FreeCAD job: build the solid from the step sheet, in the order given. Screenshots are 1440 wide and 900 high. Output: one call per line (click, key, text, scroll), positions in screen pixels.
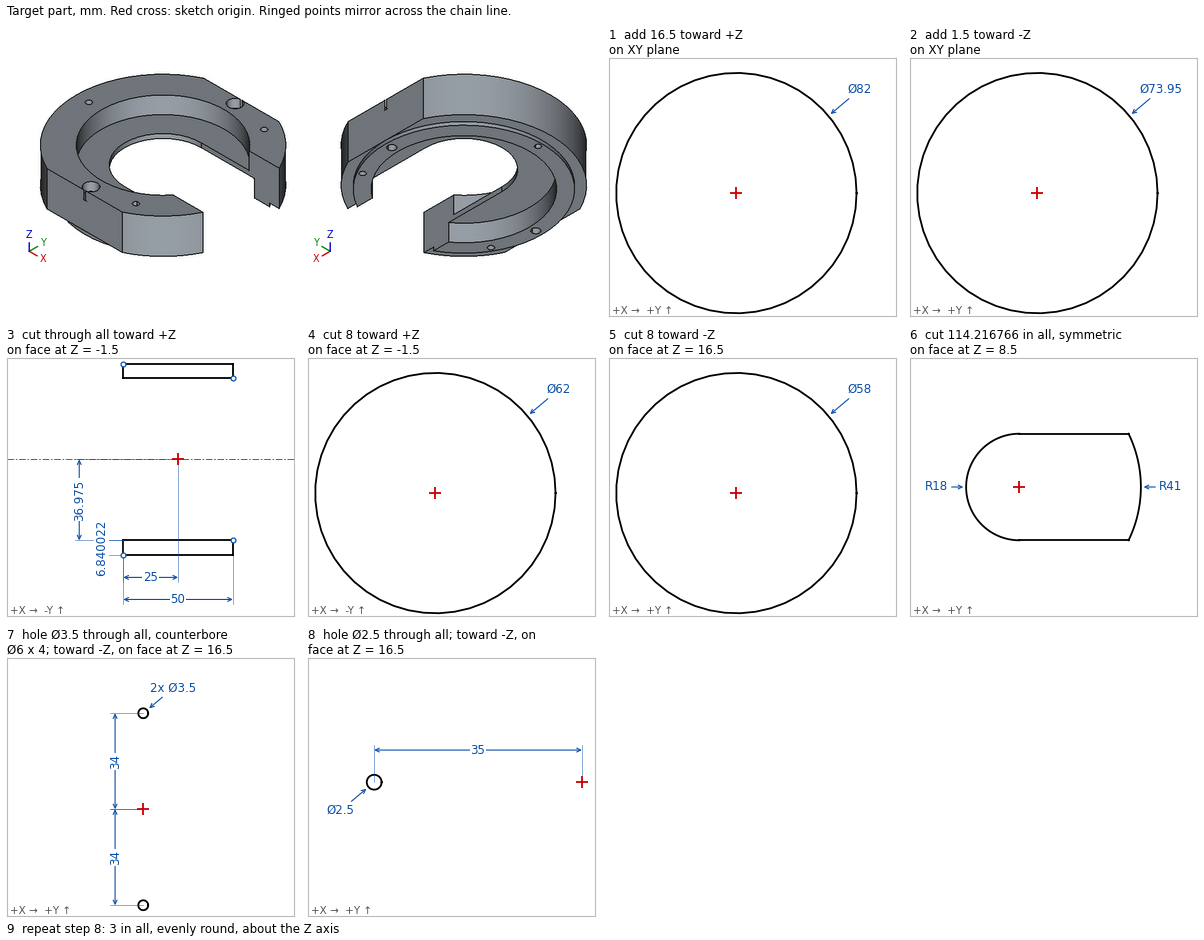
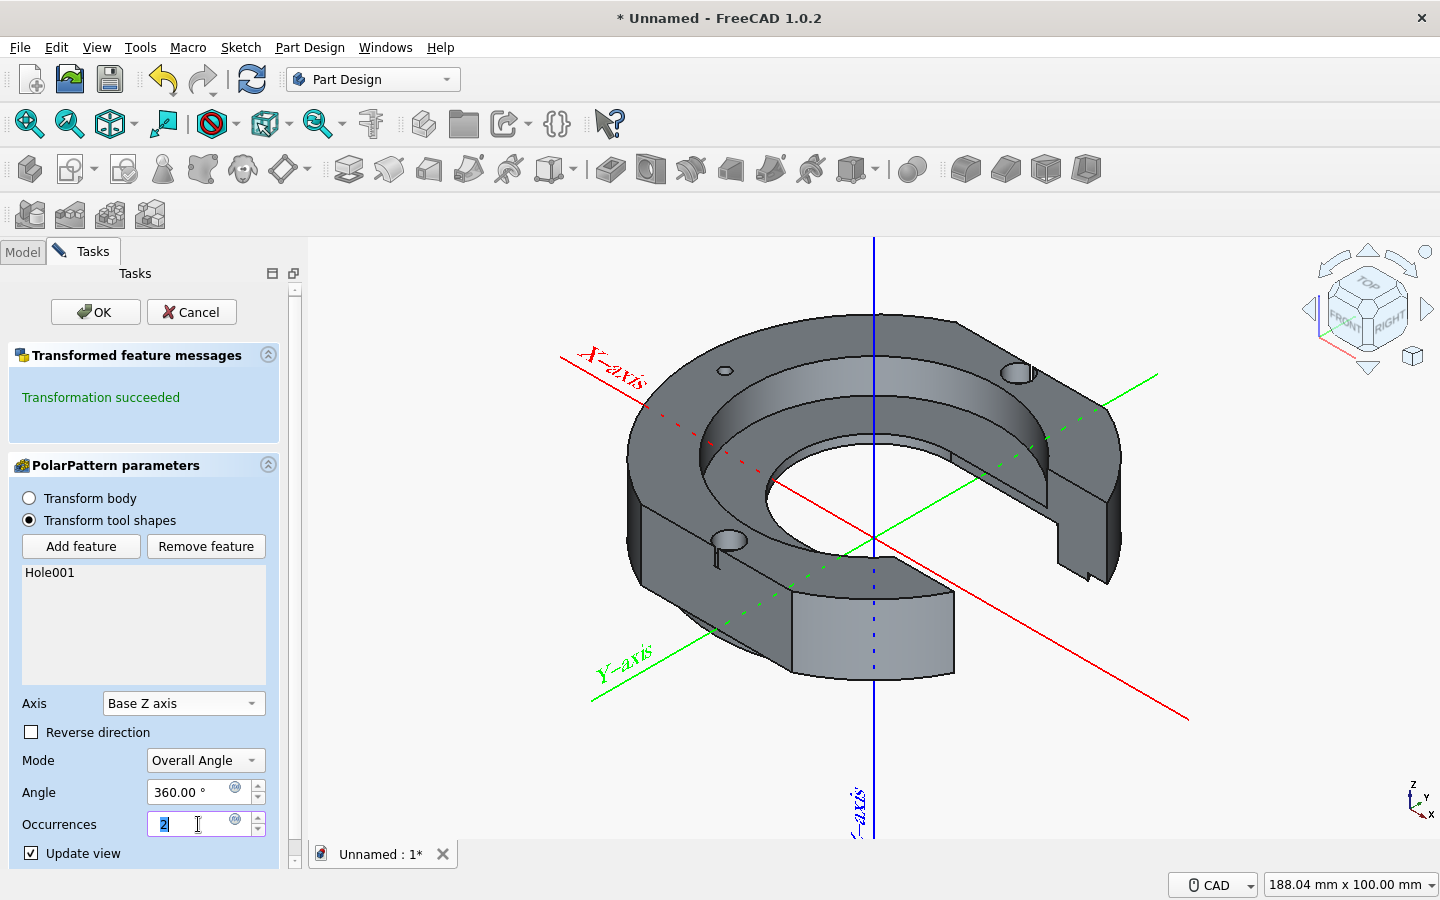
text(3)
key(Tab)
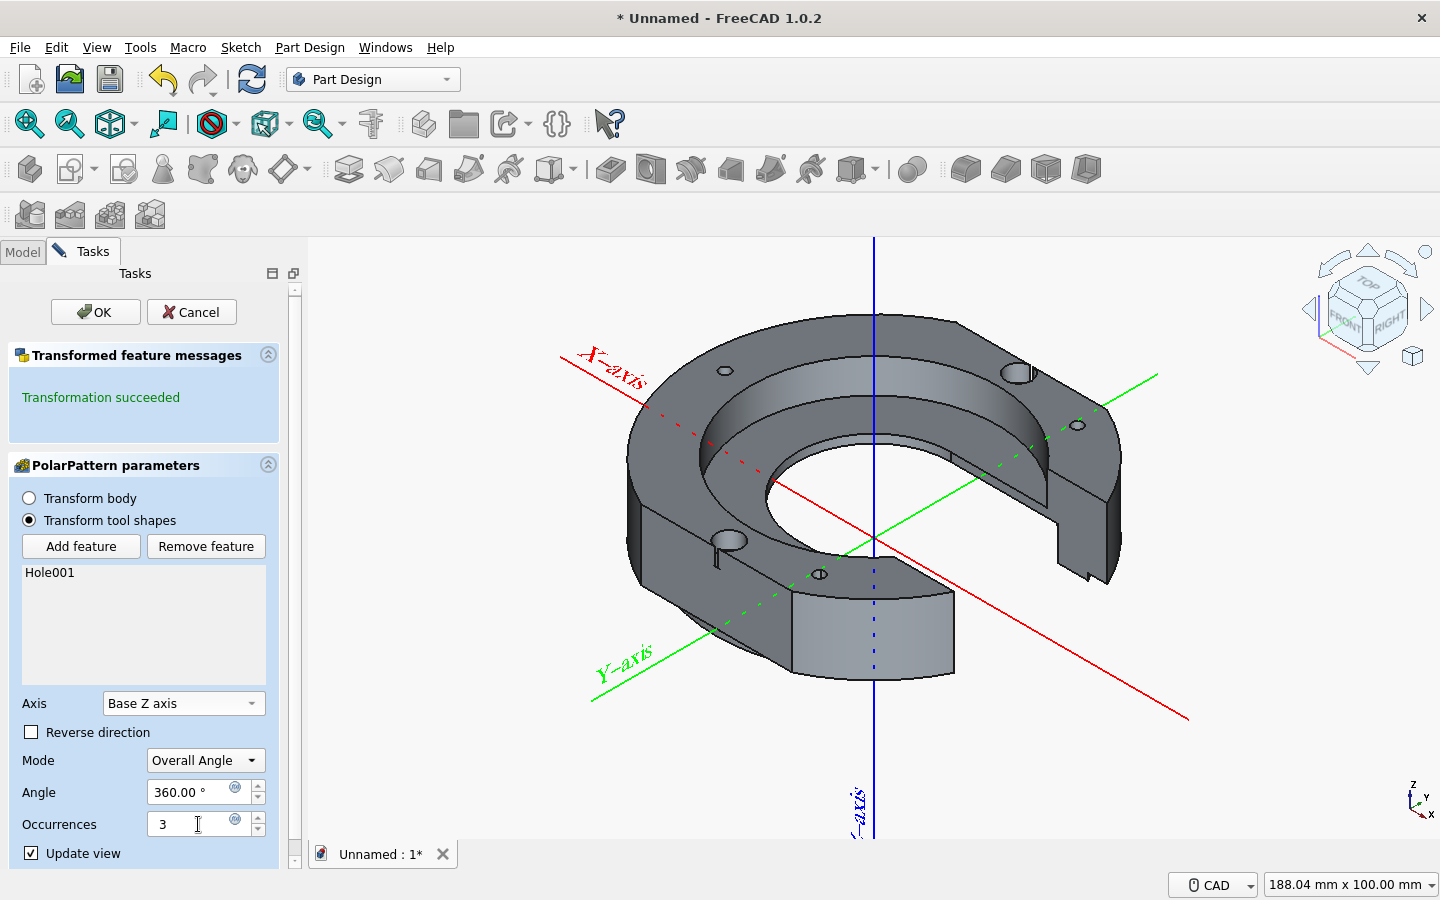
click(96, 312)